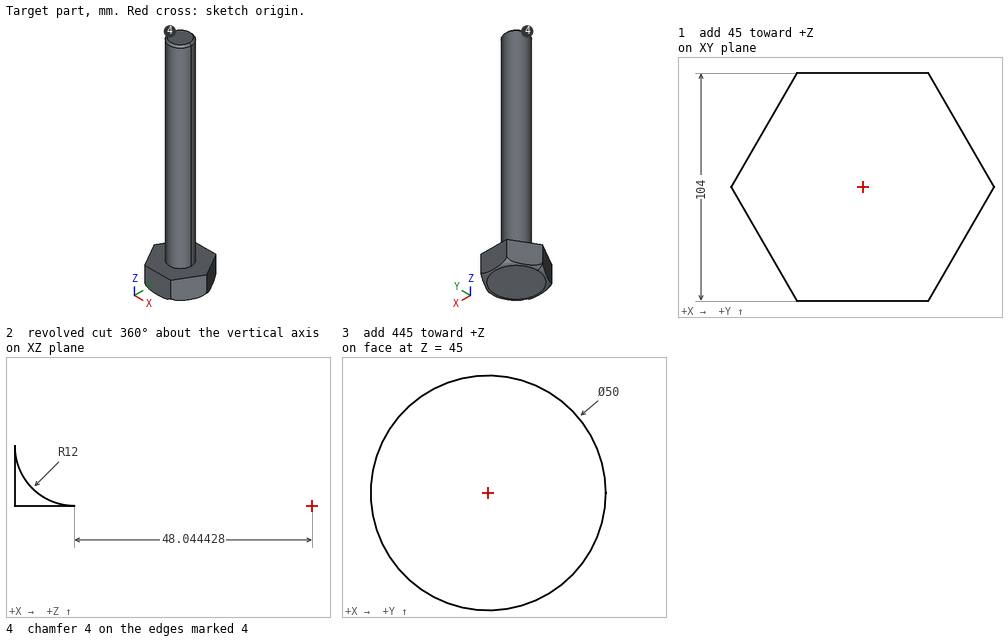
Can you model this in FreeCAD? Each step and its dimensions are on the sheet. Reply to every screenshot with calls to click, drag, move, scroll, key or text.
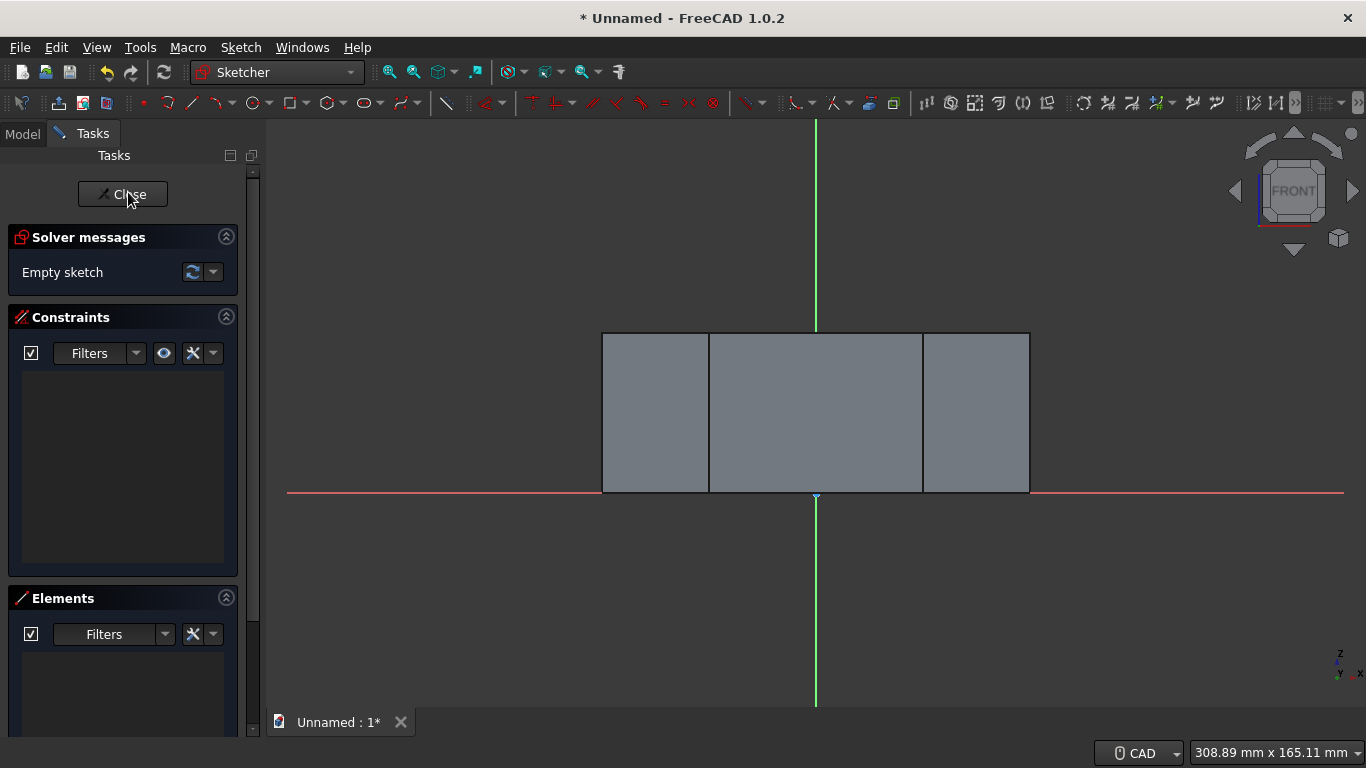
click(108, 104)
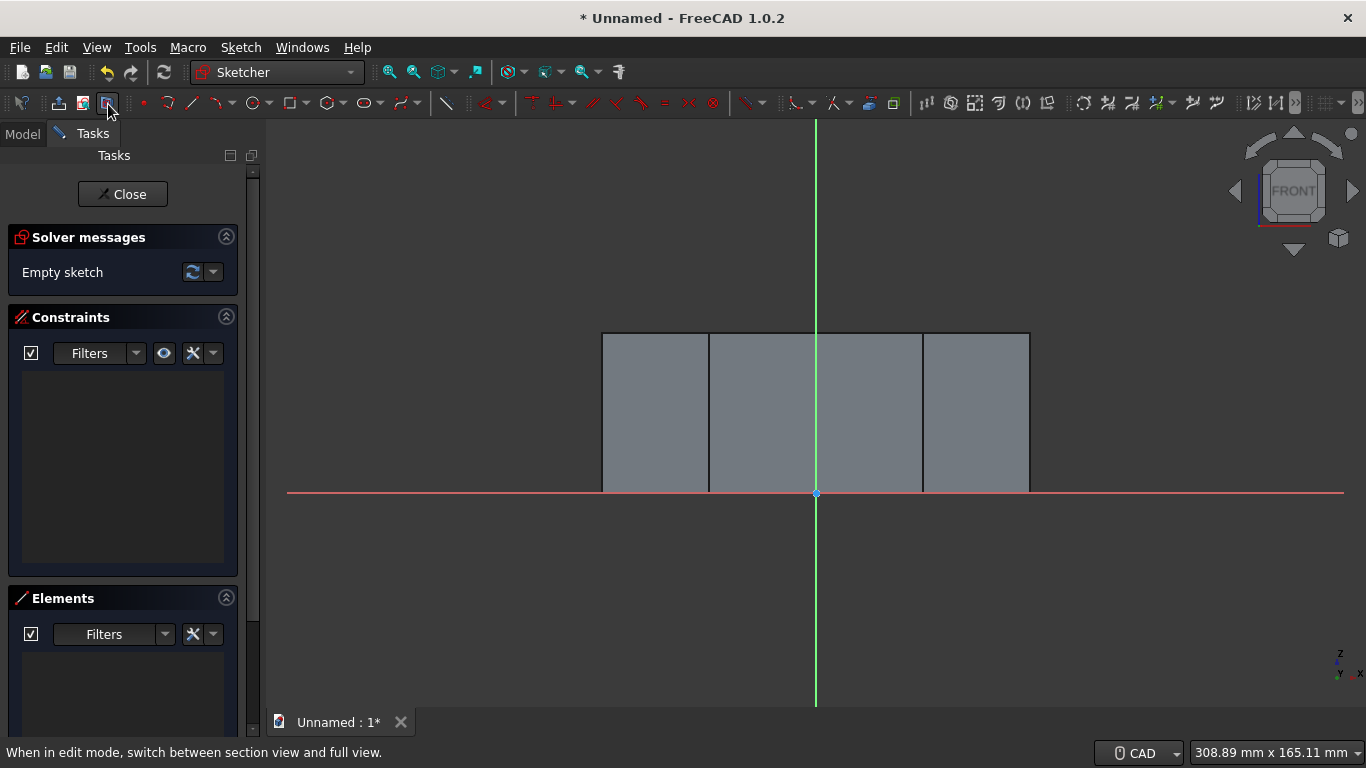
scroll(608, 479, up, 11)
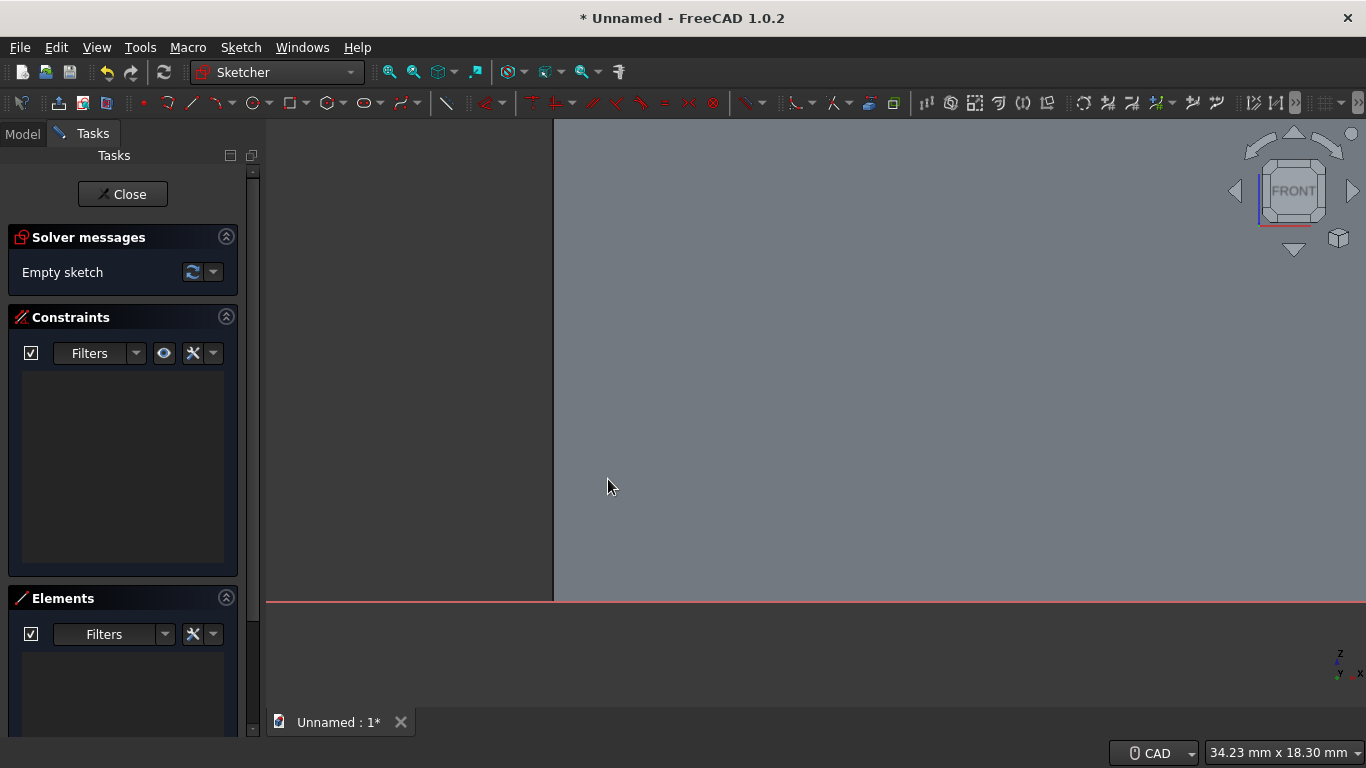
key(g)
key(m)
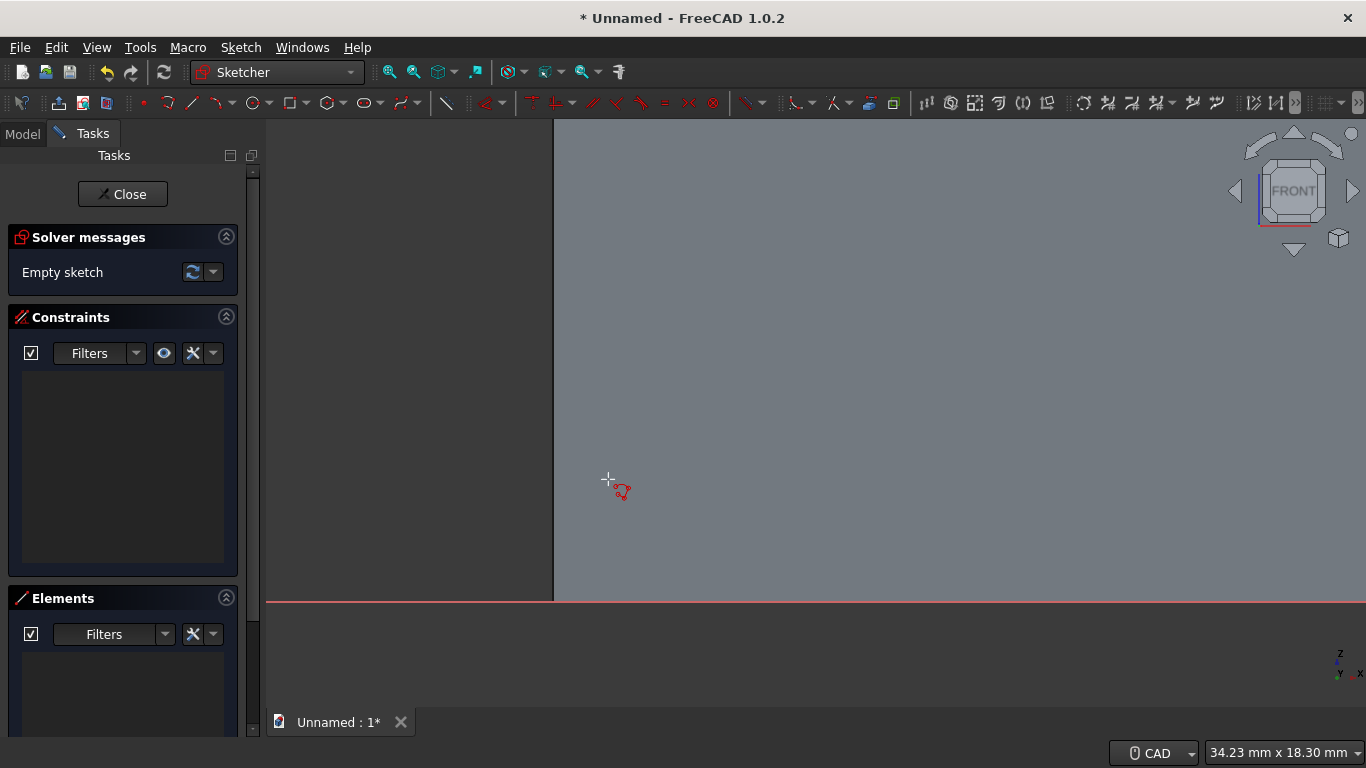
click(939, 602)
click(553, 593)
click(553, 216)
right_click(553, 216)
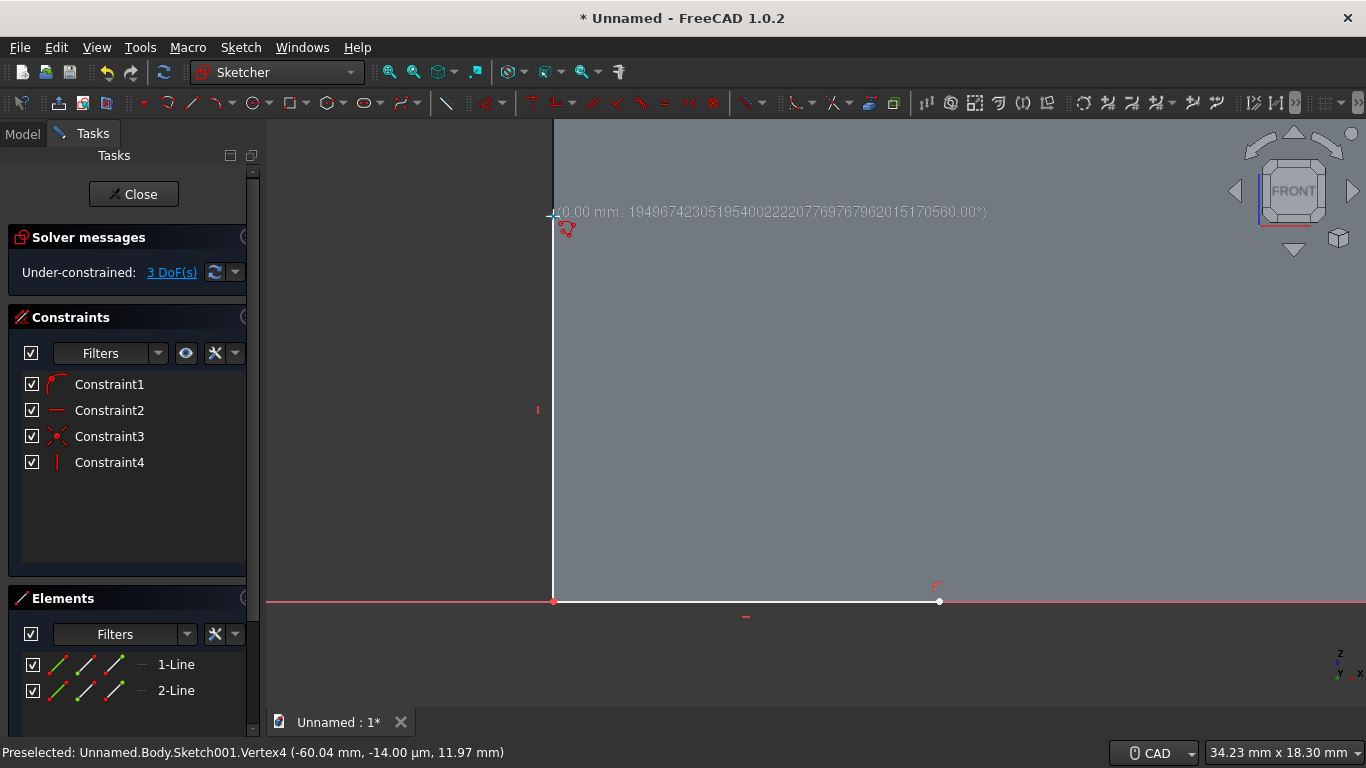
click(216, 104)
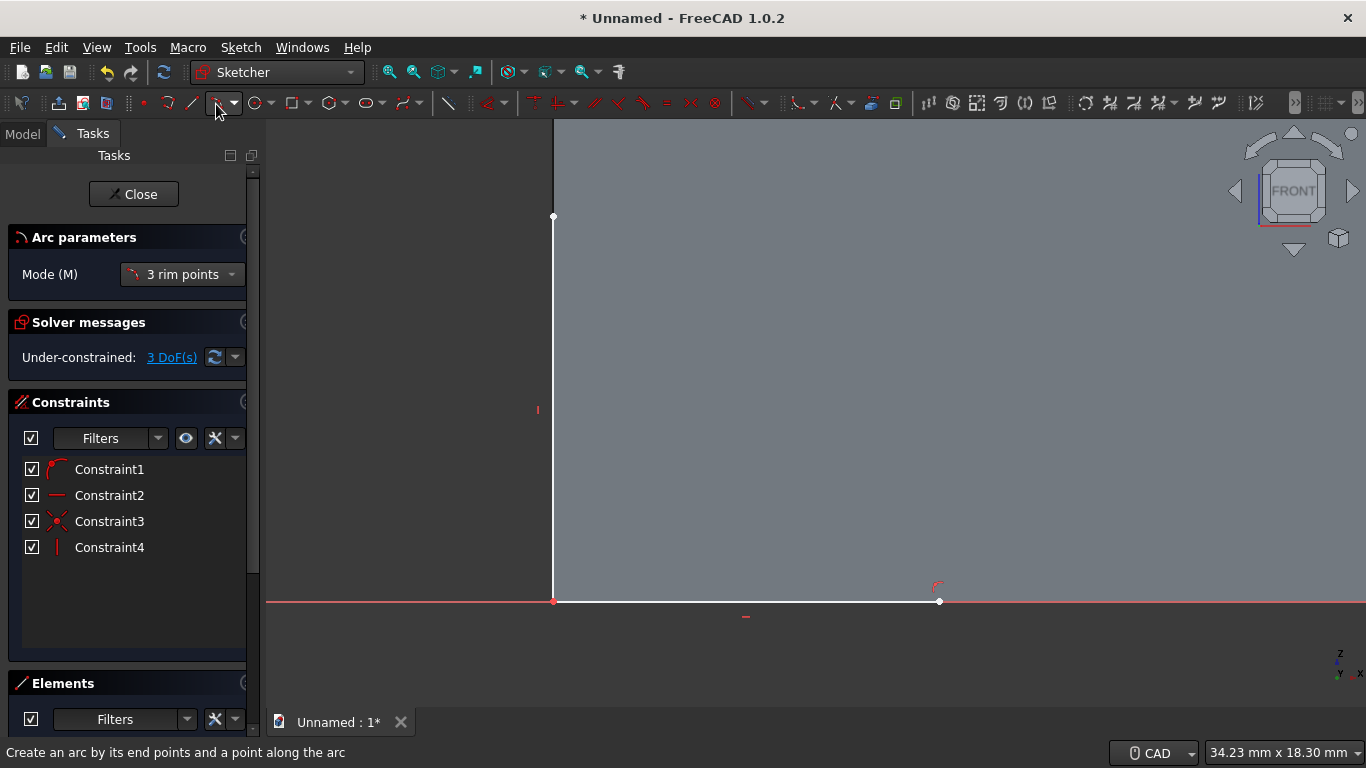
click(553, 217)
click(939, 602)
click(666, 489)
key(Escape)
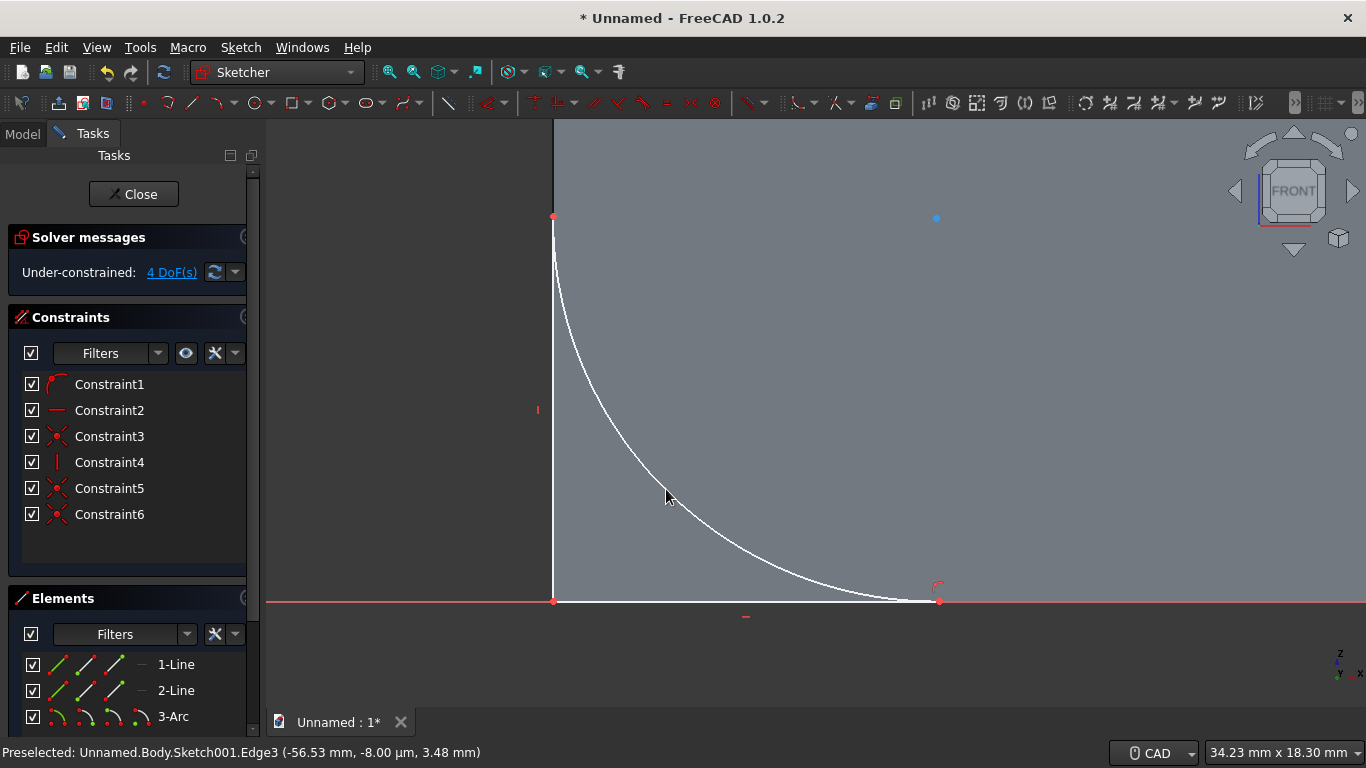
click(823, 602)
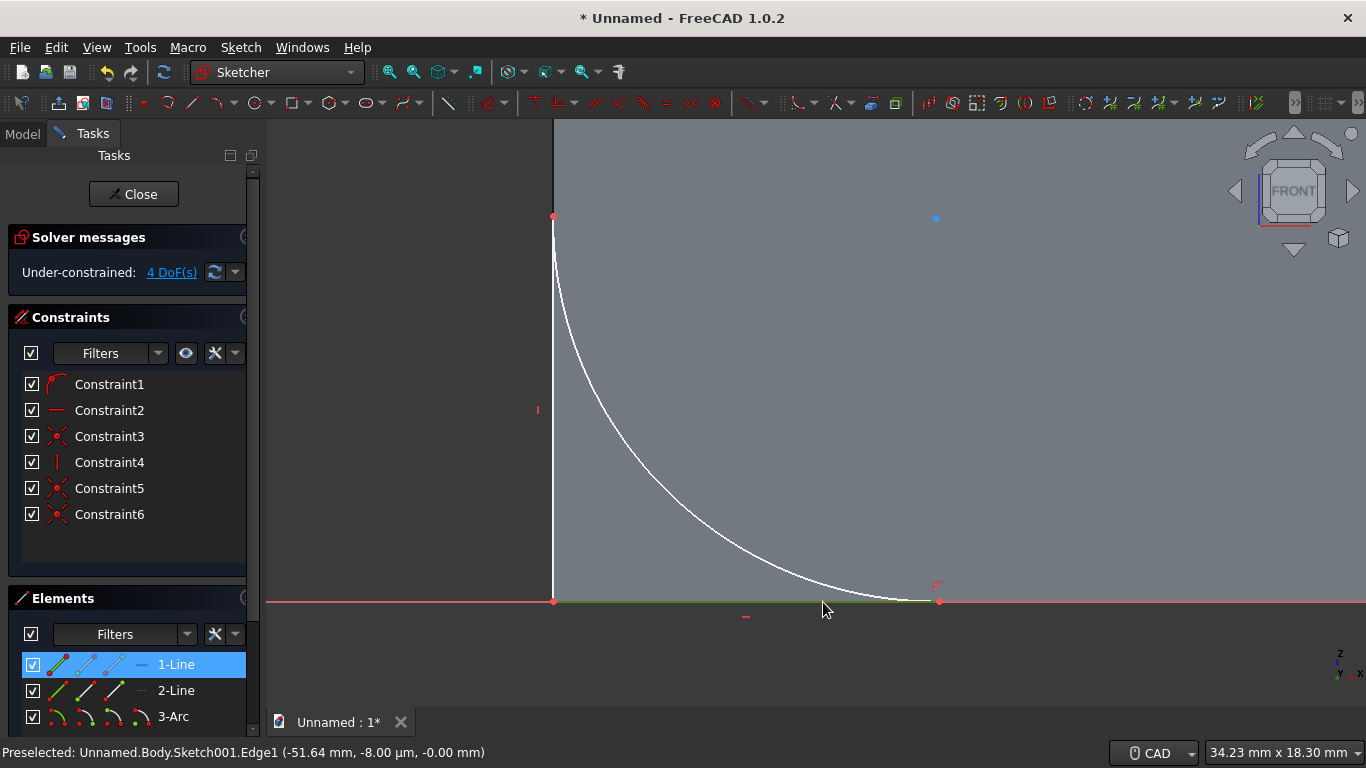
click(595, 392)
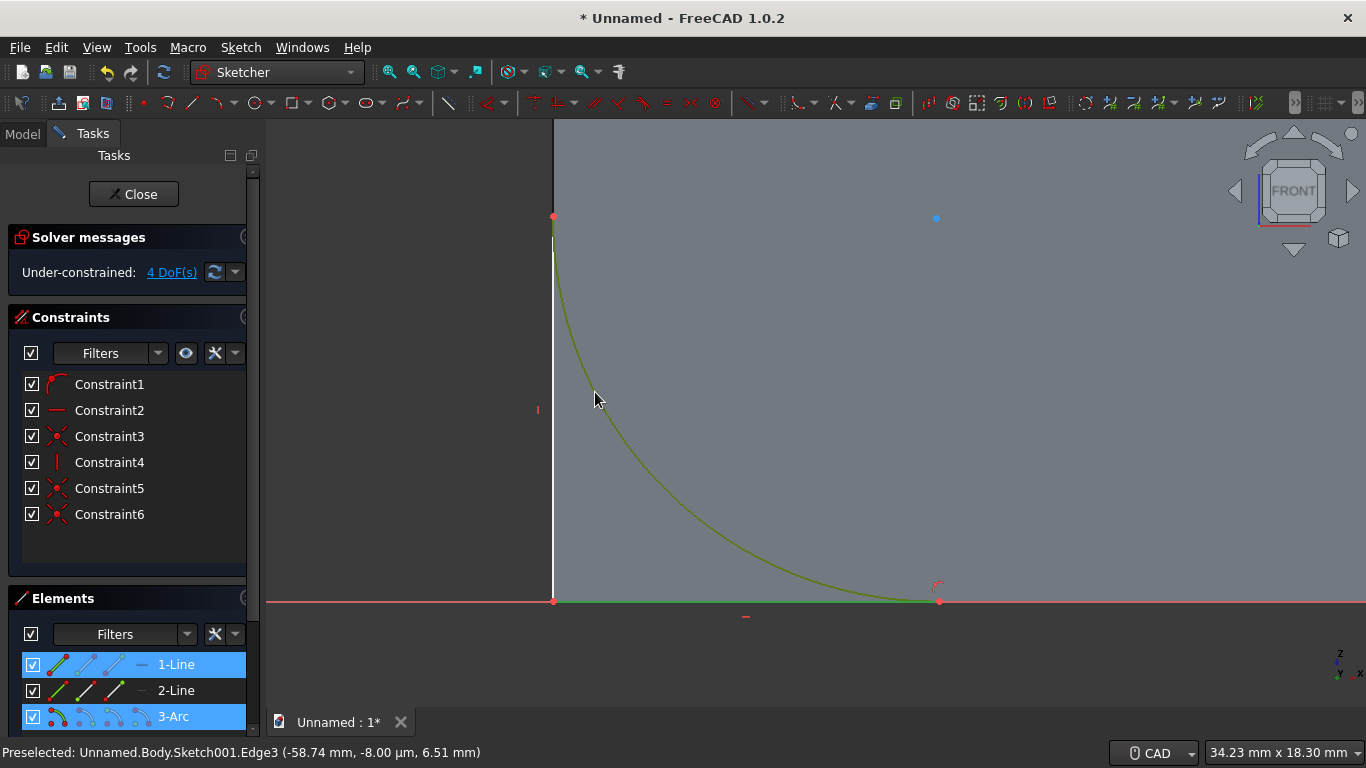
key(t)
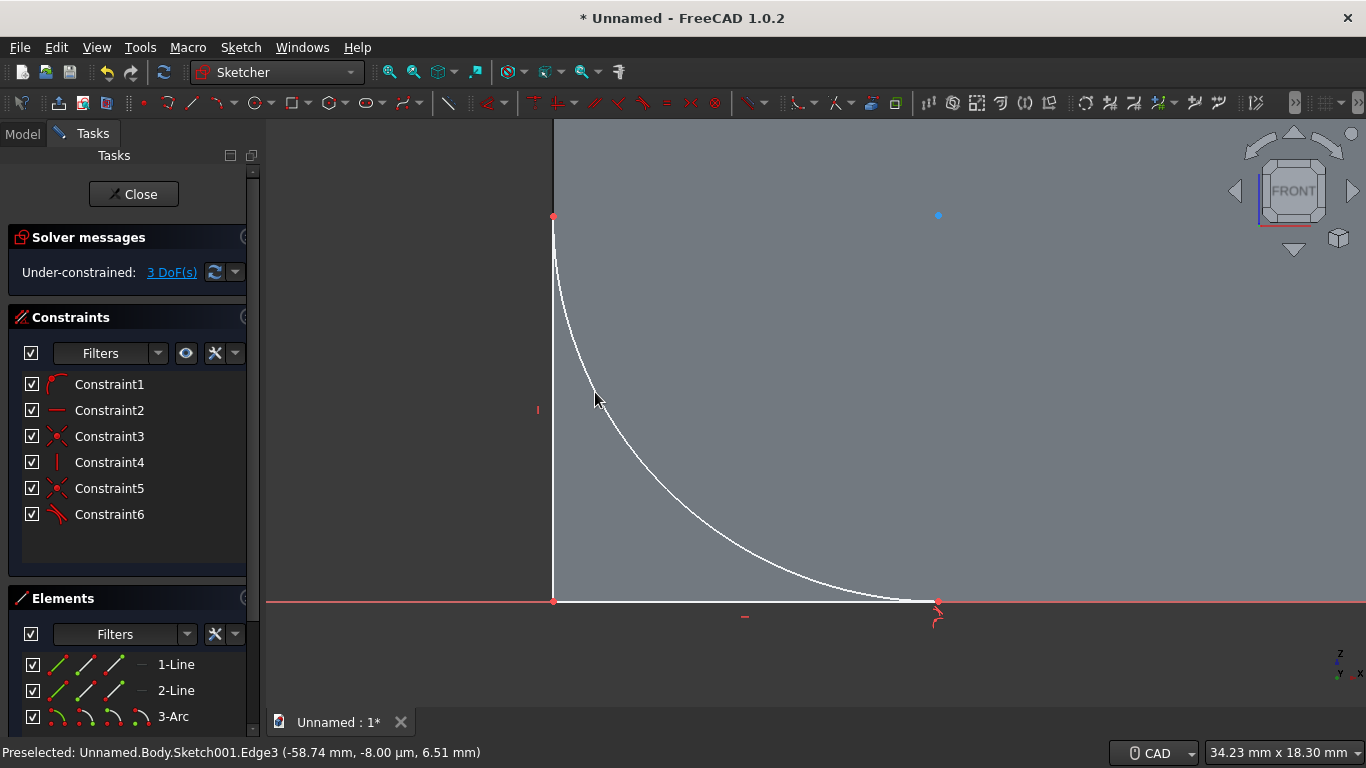
click(553, 486)